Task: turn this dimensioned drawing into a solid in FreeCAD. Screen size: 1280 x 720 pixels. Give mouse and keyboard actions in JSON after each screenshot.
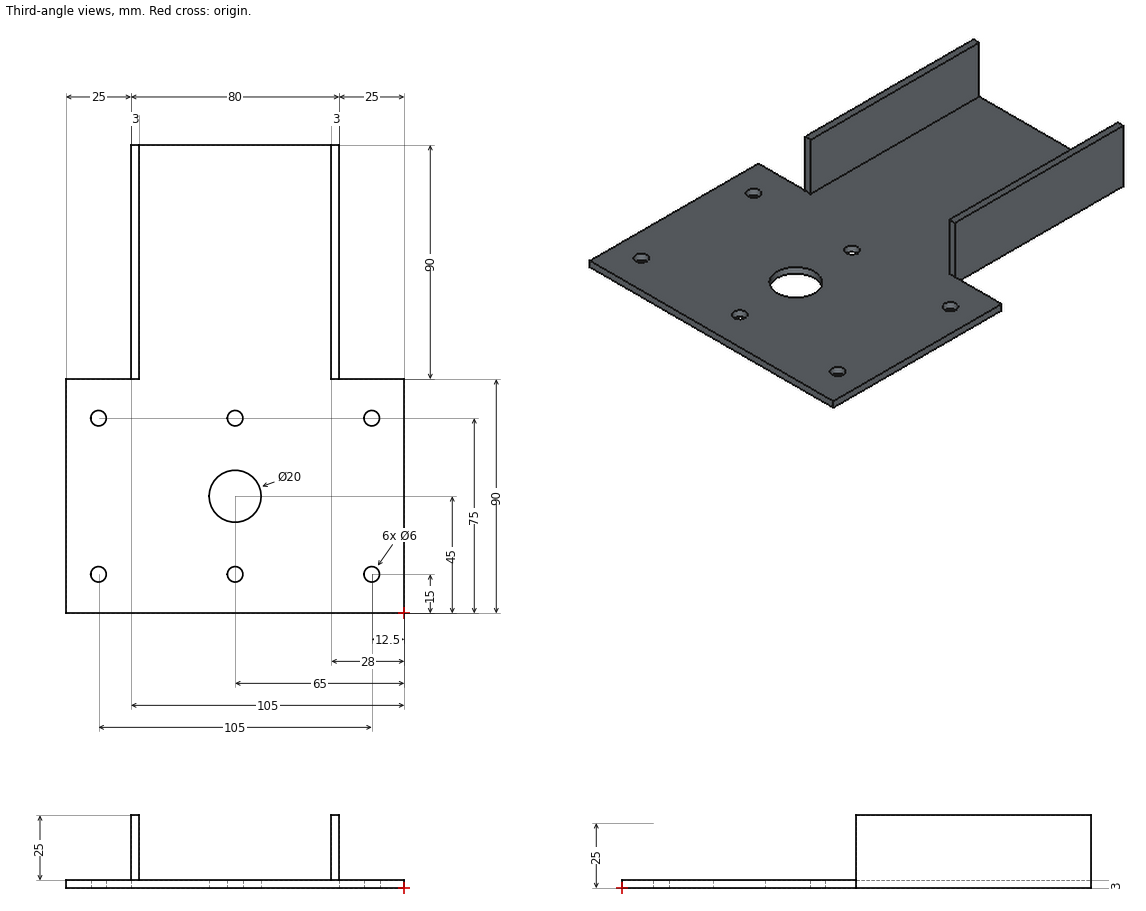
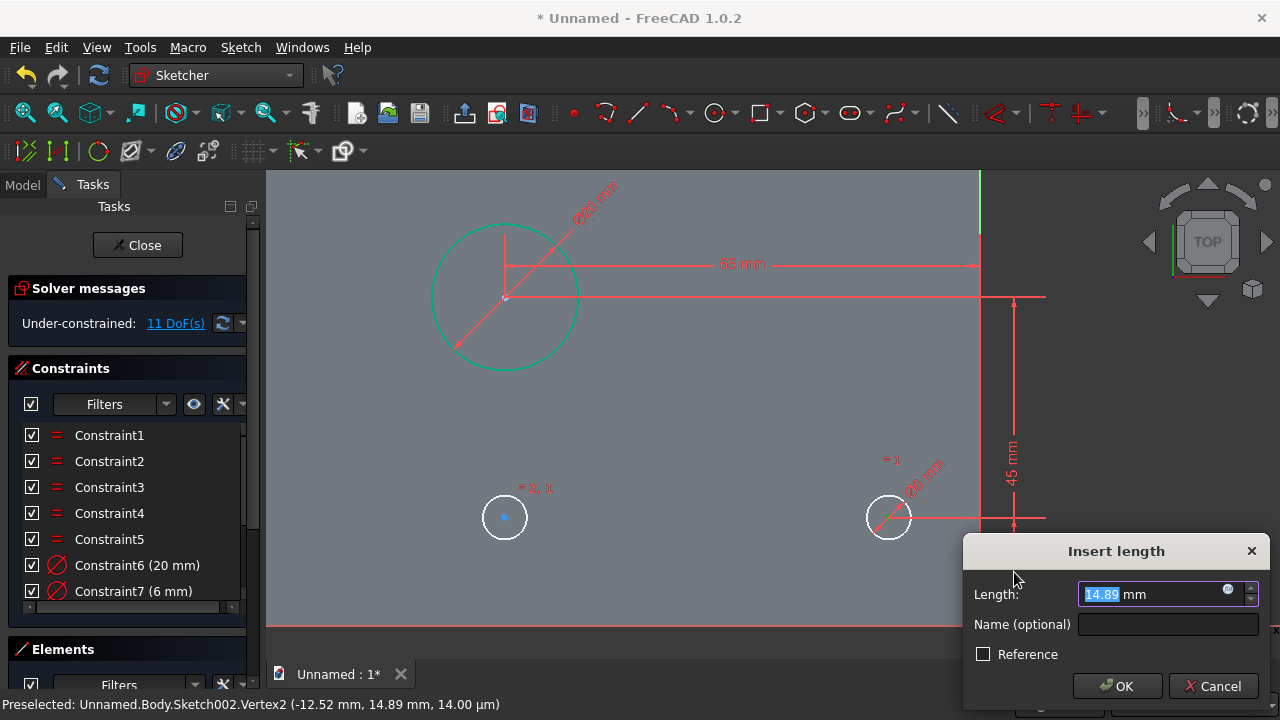
{"action": "type", "text": "15"}
{"action": "key", "text": "Return"}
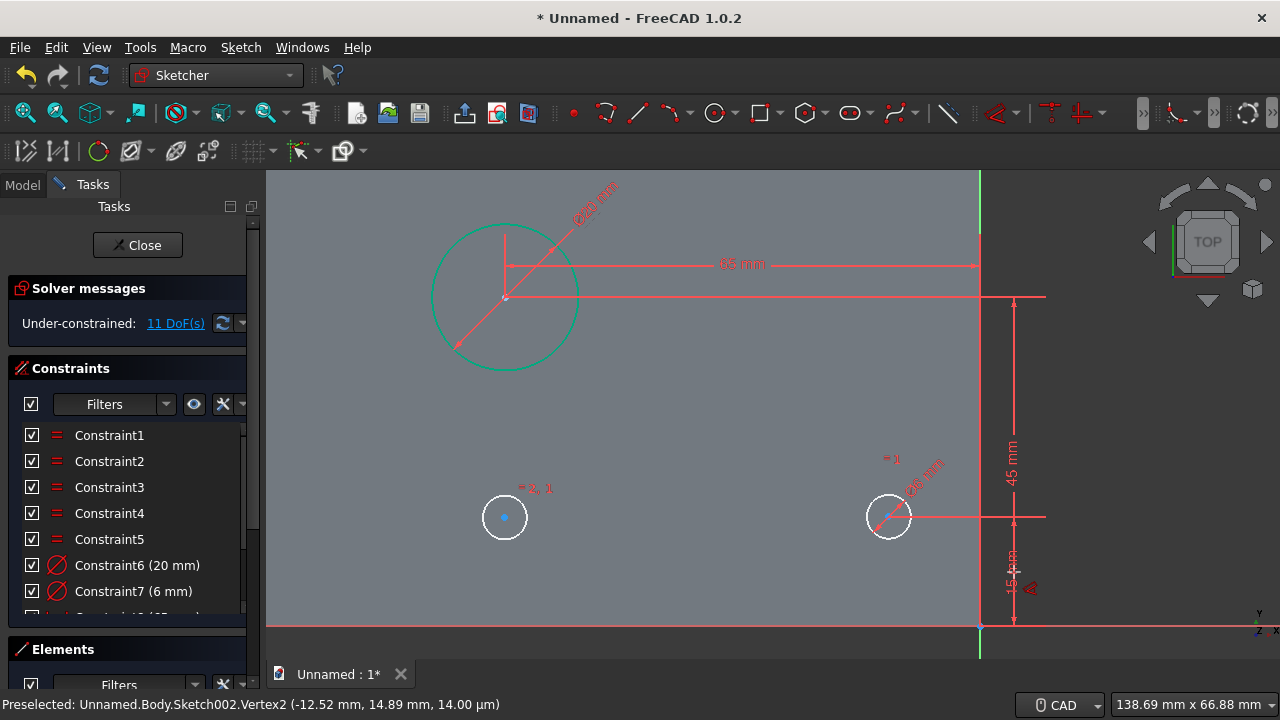
{"action": "left_click", "coordinate": [505, 518]}
{"action": "left_click", "coordinate": [743, 484]}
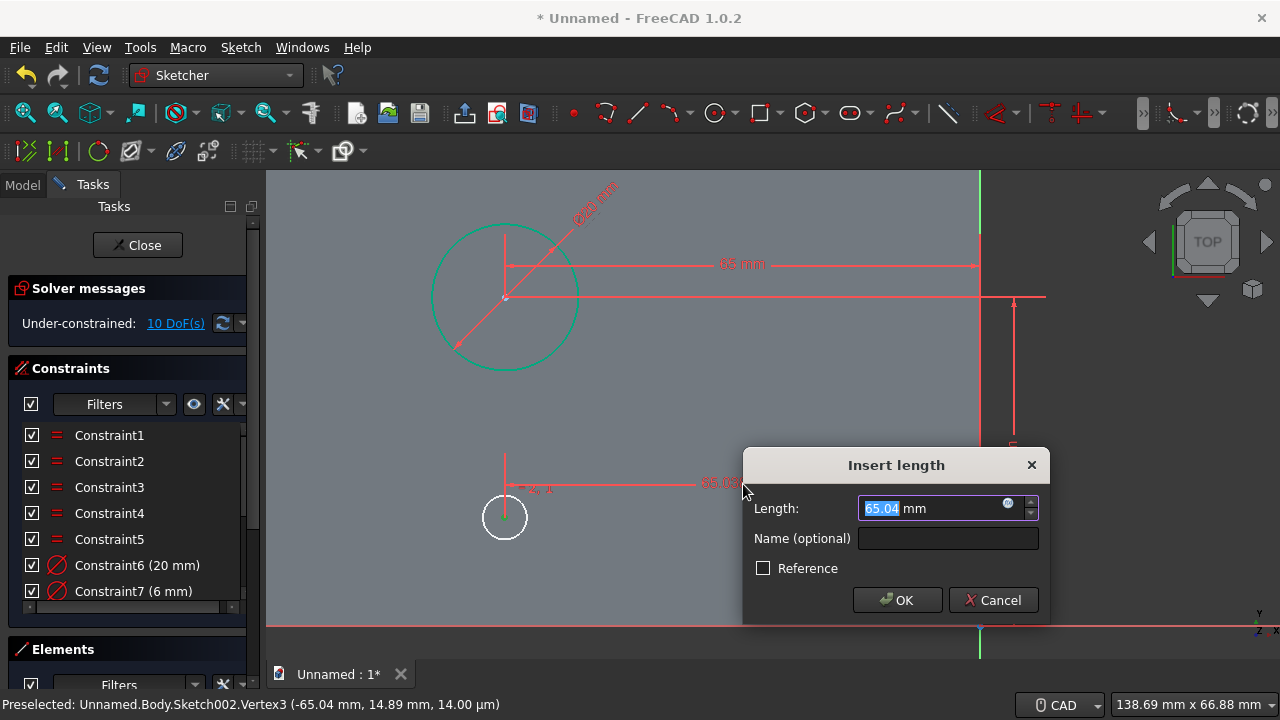
{"action": "type", "text": "65"}
{"action": "key", "text": "Return"}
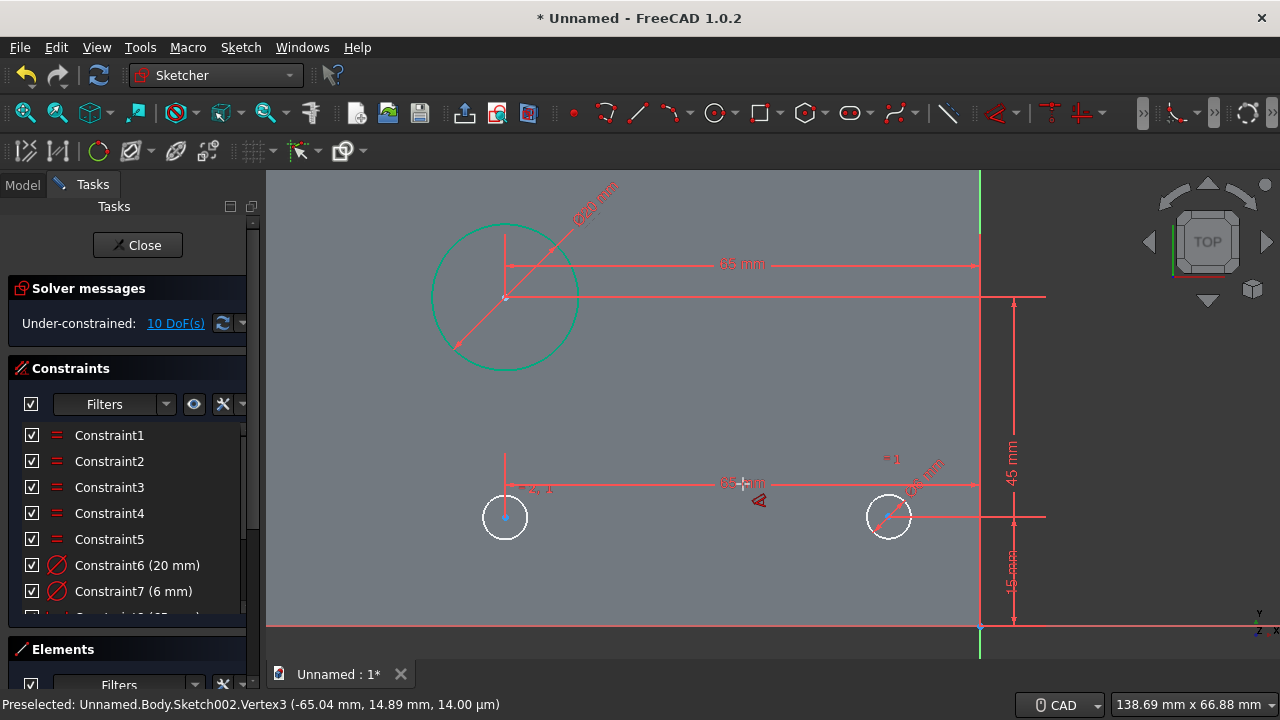
{"action": "left_click", "coordinate": [505, 518]}
{"action": "left_click", "coordinate": [1014, 547]}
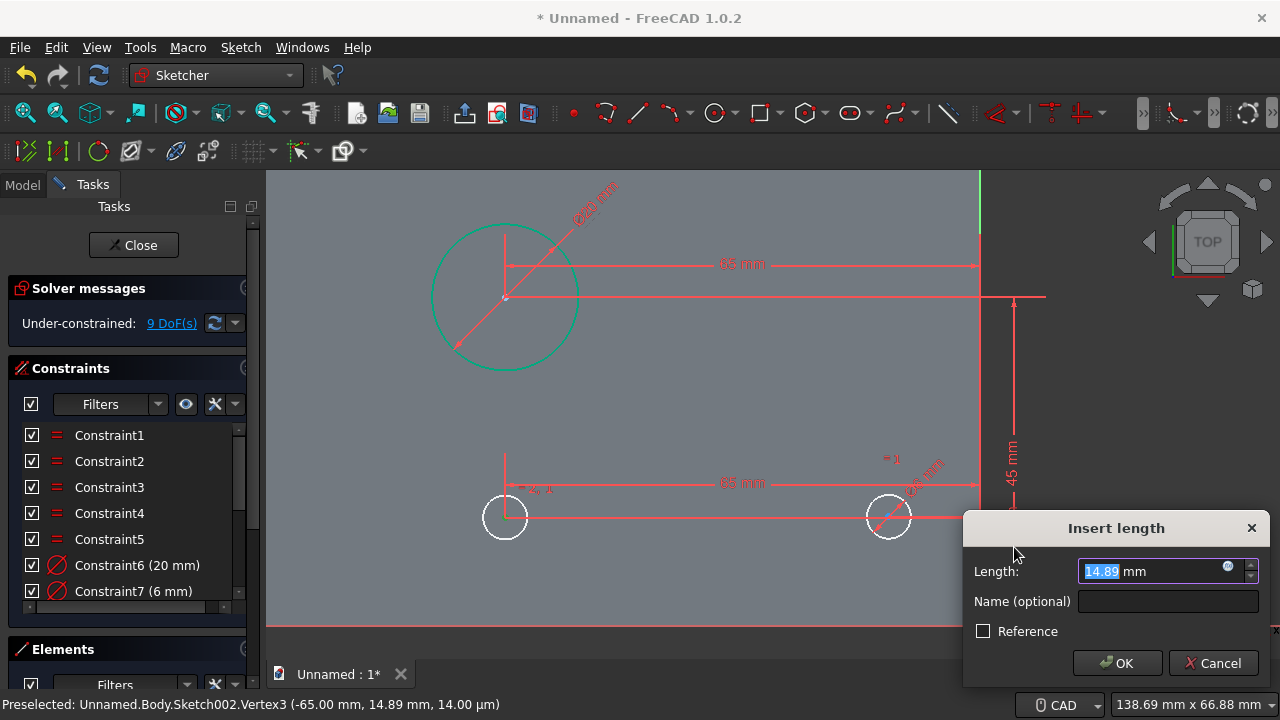
{"action": "type", "text": "15"}
{"action": "key", "text": "Return"}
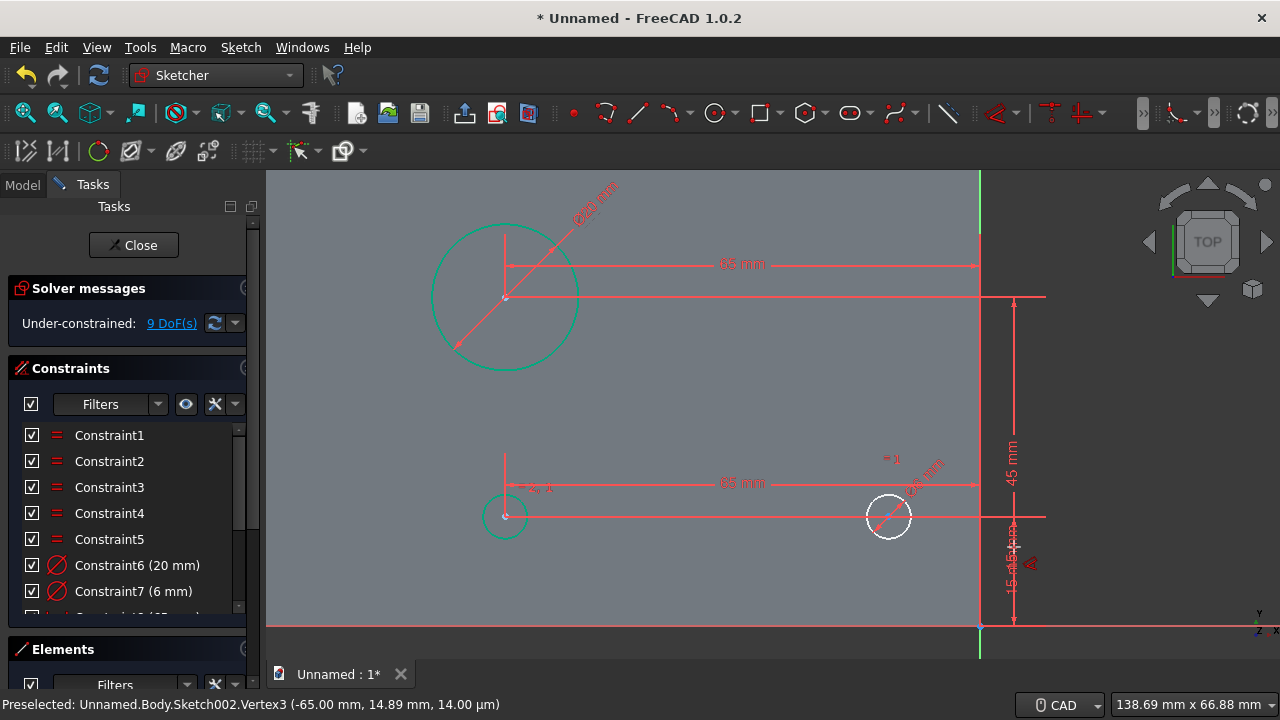
{"action": "scroll", "coordinate": [905, 504], "scroll_direction": "down", "scroll_amount": 3}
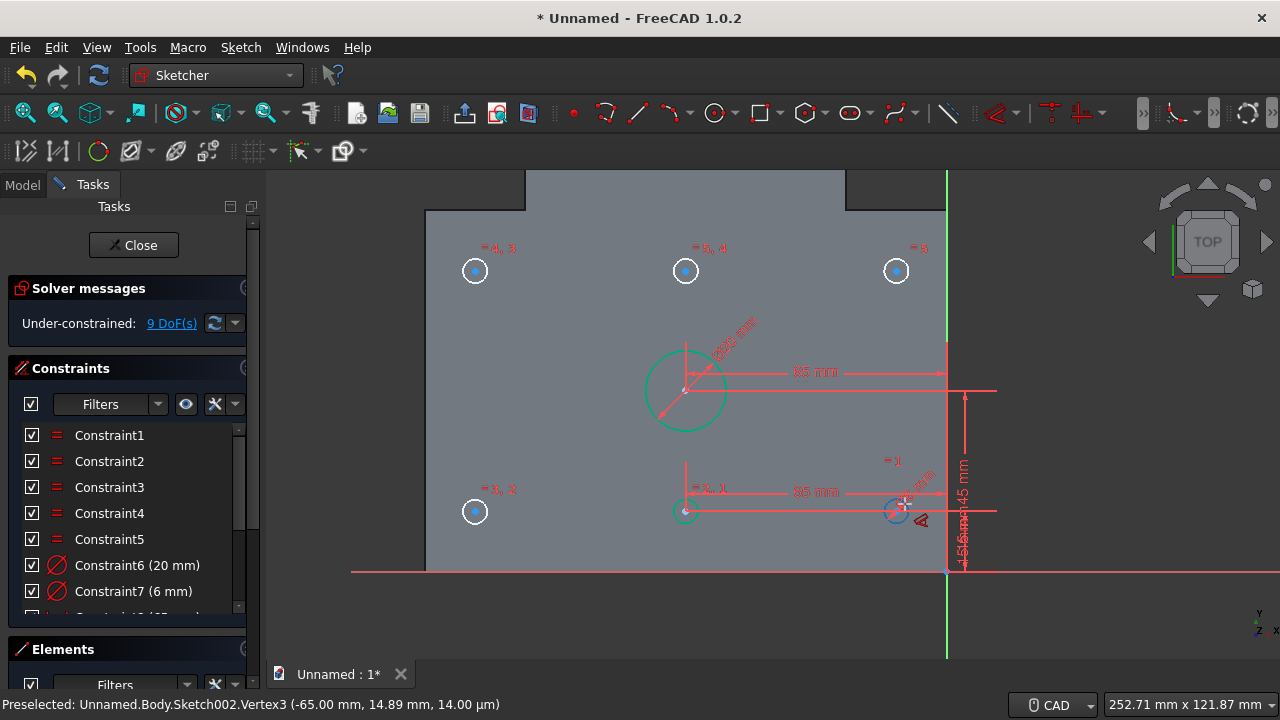
{"action": "left_click", "coordinate": [475, 512]}
{"action": "left_click", "coordinate": [441, 542]}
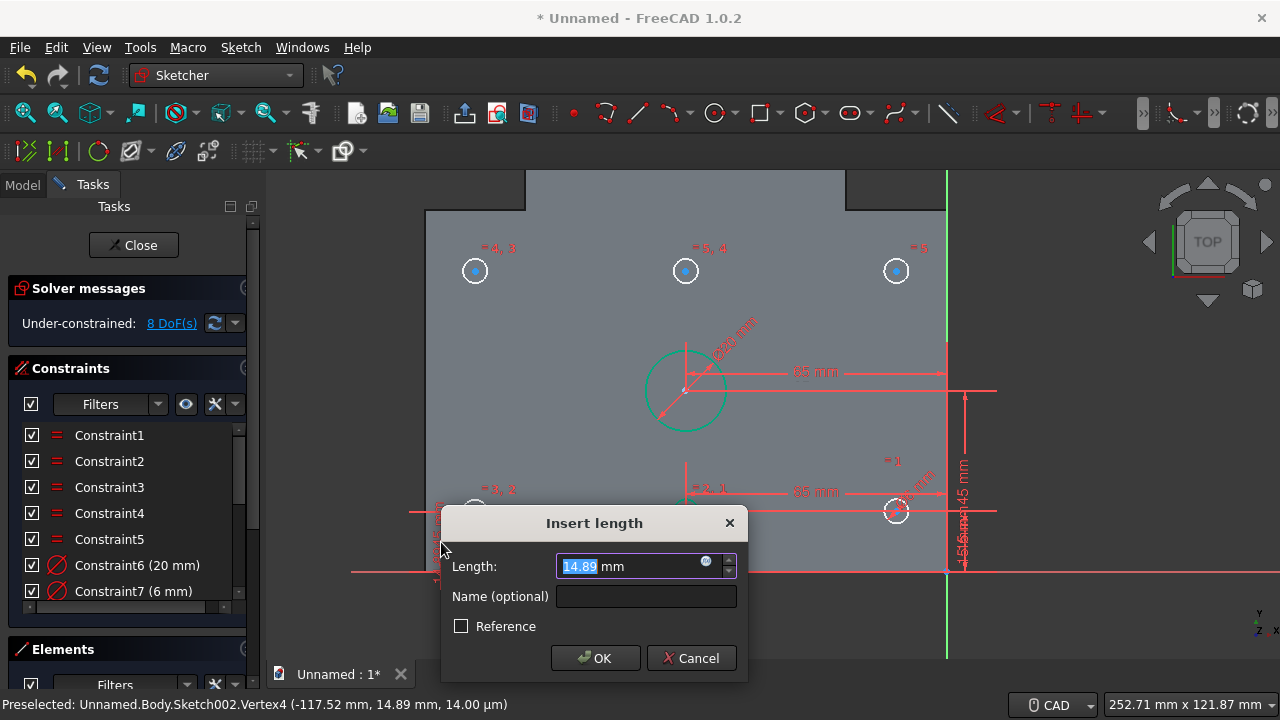
{"action": "type", "text": "15"}
{"action": "key", "text": "Return"}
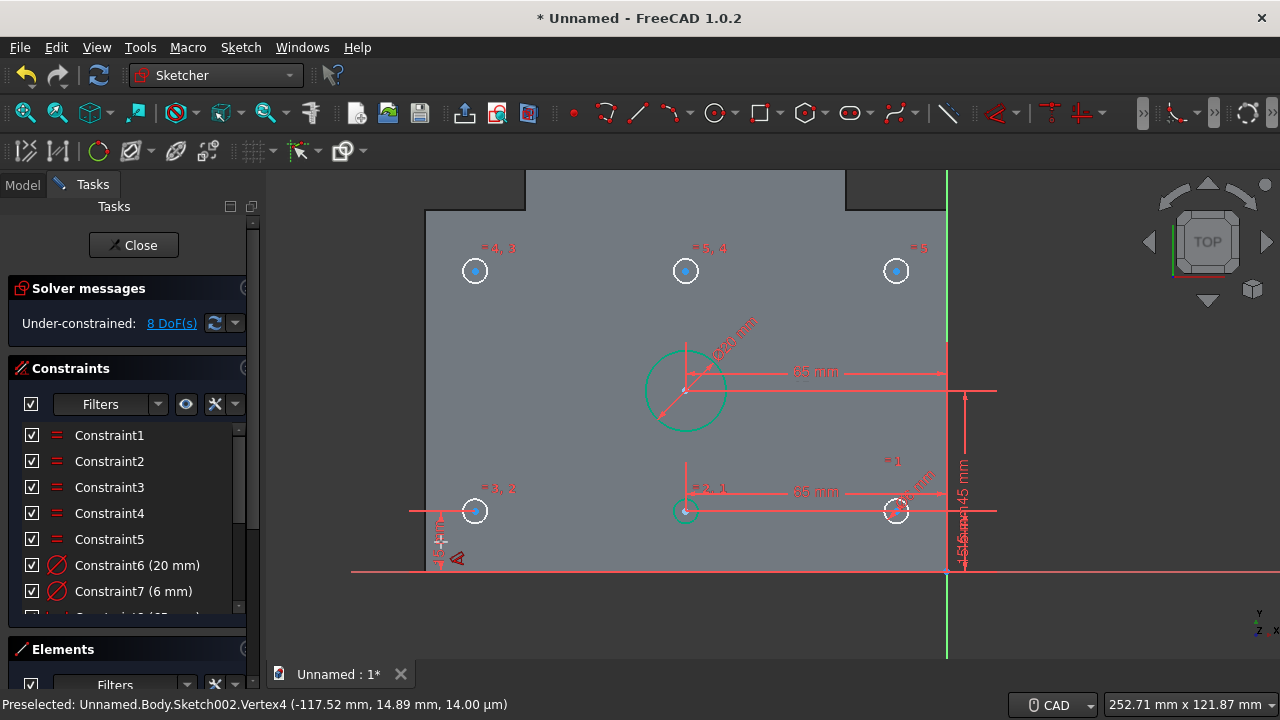
{"action": "left_click", "coordinate": [475, 271]}
{"action": "left_click", "coordinate": [981, 421]}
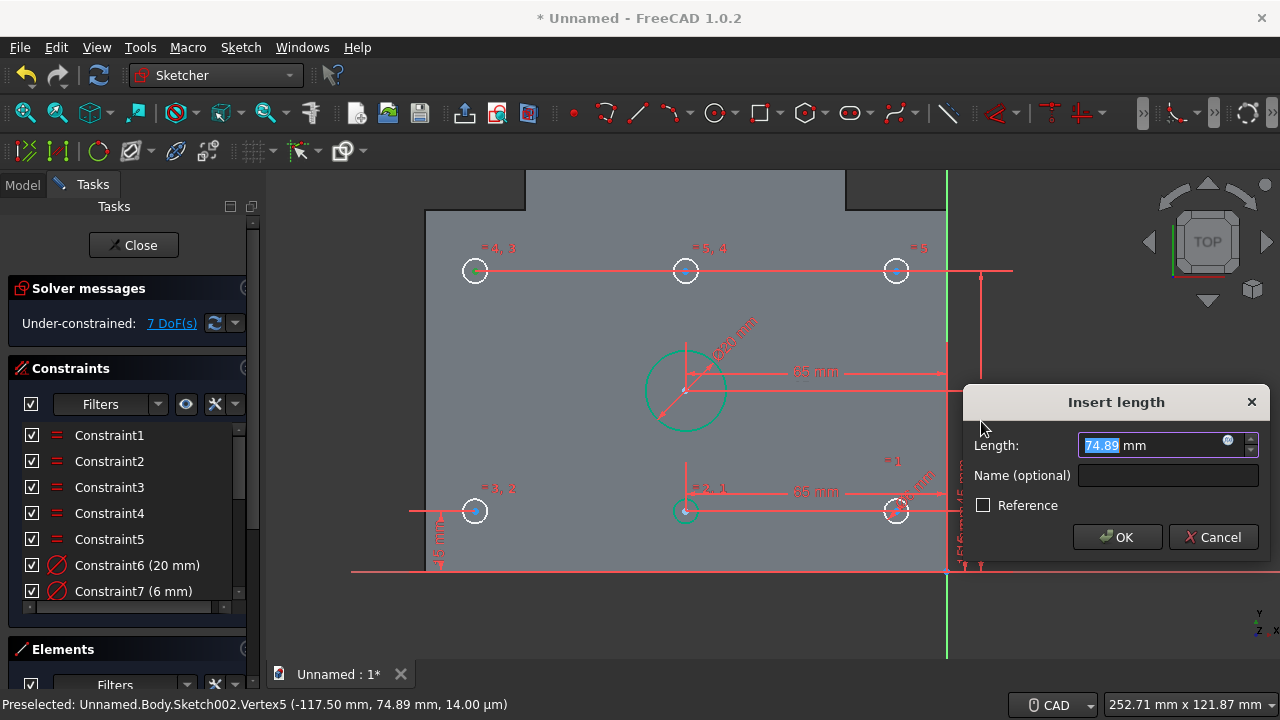
{"action": "type", "text": "75"}
{"action": "key", "text": "Return"}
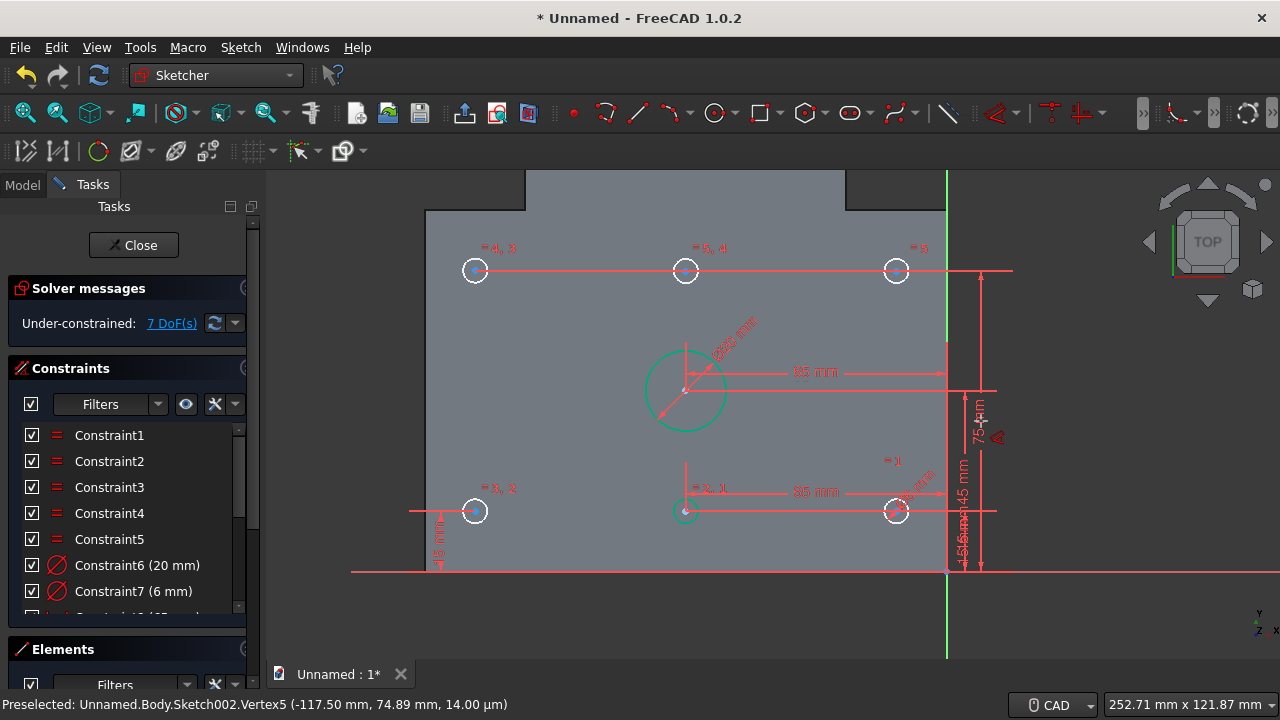
{"action": "left_click", "coordinate": [686, 271]}
{"action": "left_click", "coordinate": [816, 605]}